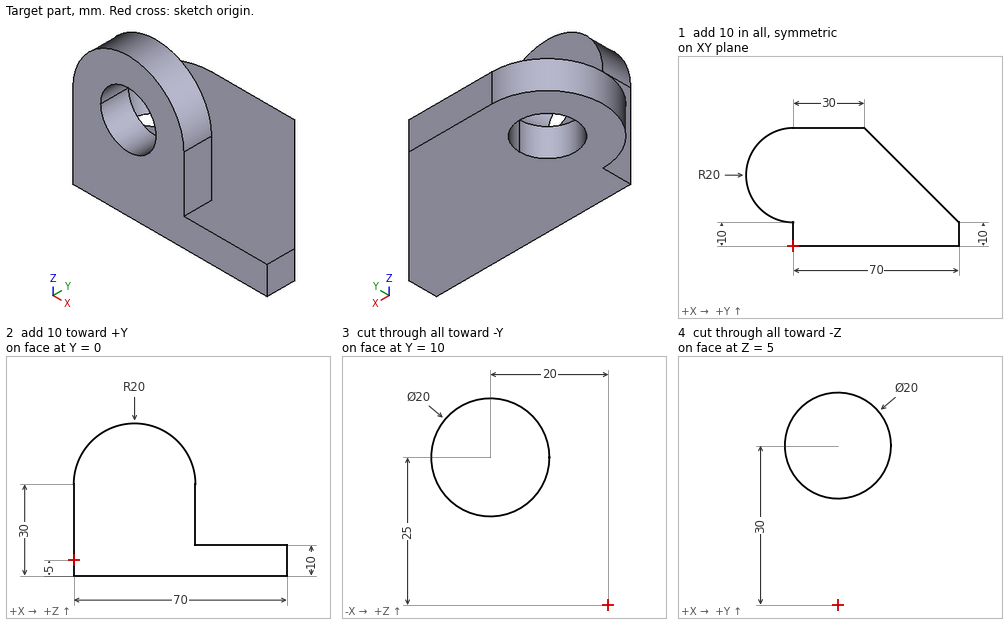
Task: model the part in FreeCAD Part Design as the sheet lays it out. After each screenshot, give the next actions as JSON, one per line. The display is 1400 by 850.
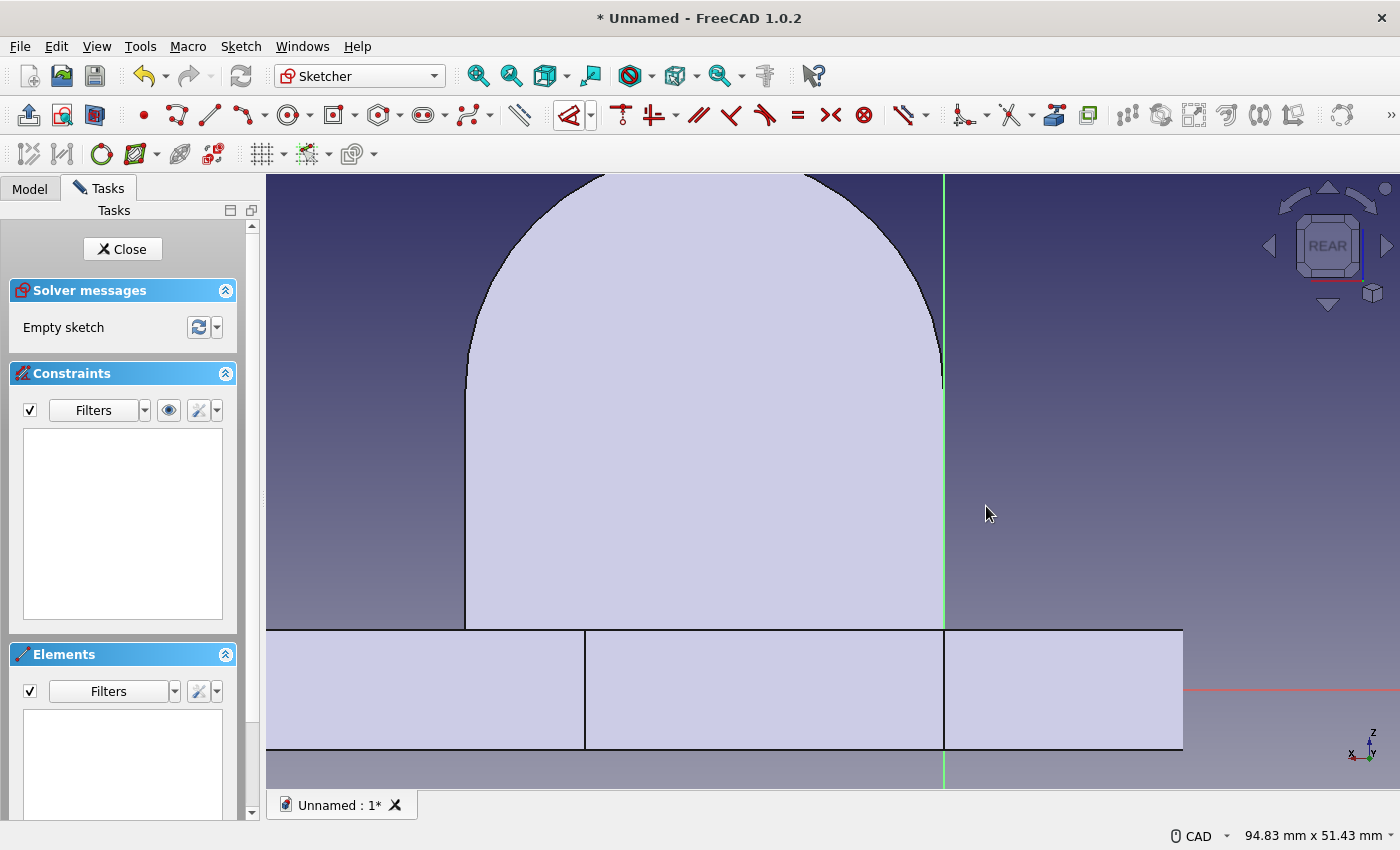
{"action": "left_click", "coordinate": [288, 116]}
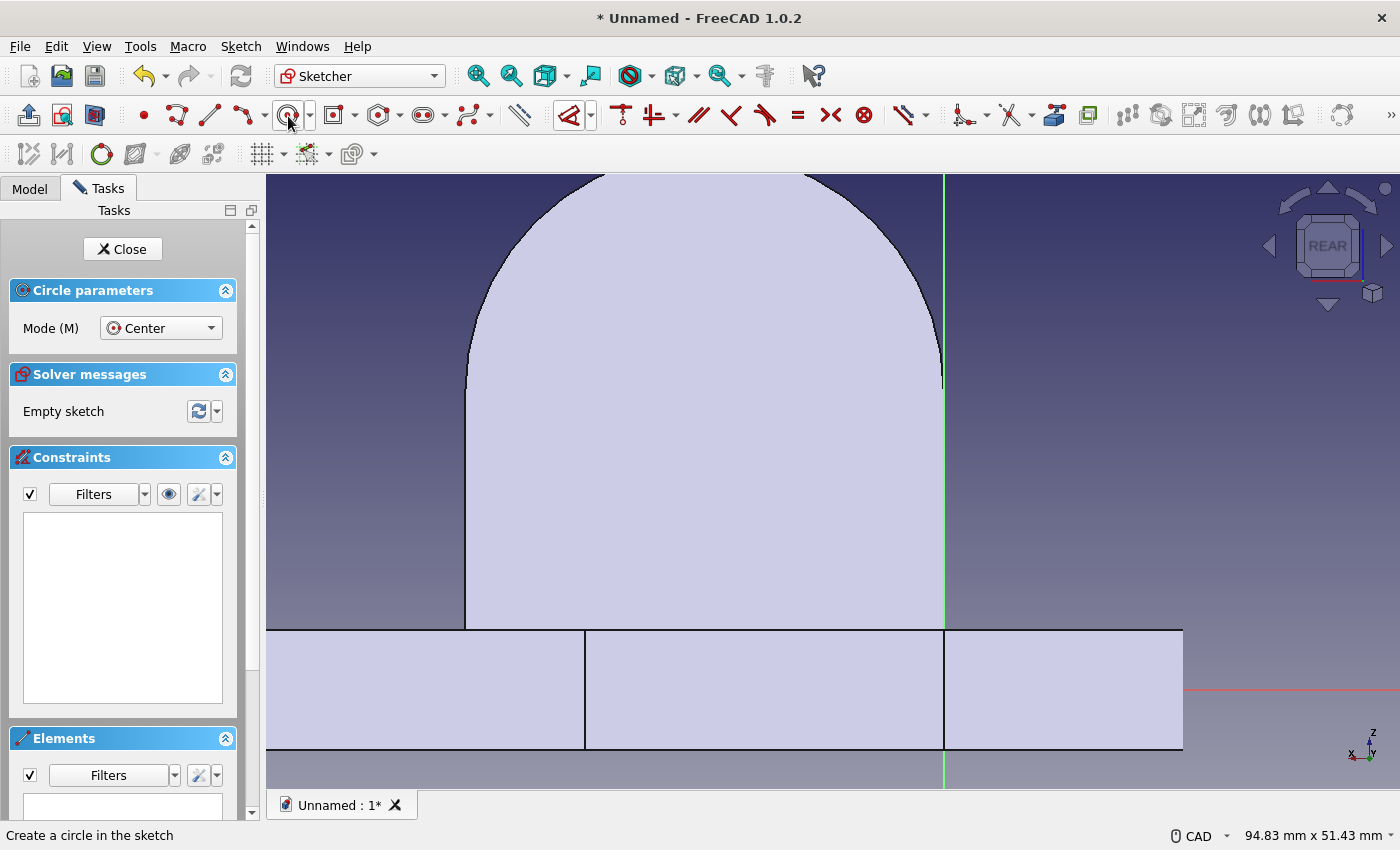
{"action": "left_click", "coordinate": [705, 391]}
{"action": "left_click", "coordinate": [789, 306]}
{"action": "key", "text": "Escape"}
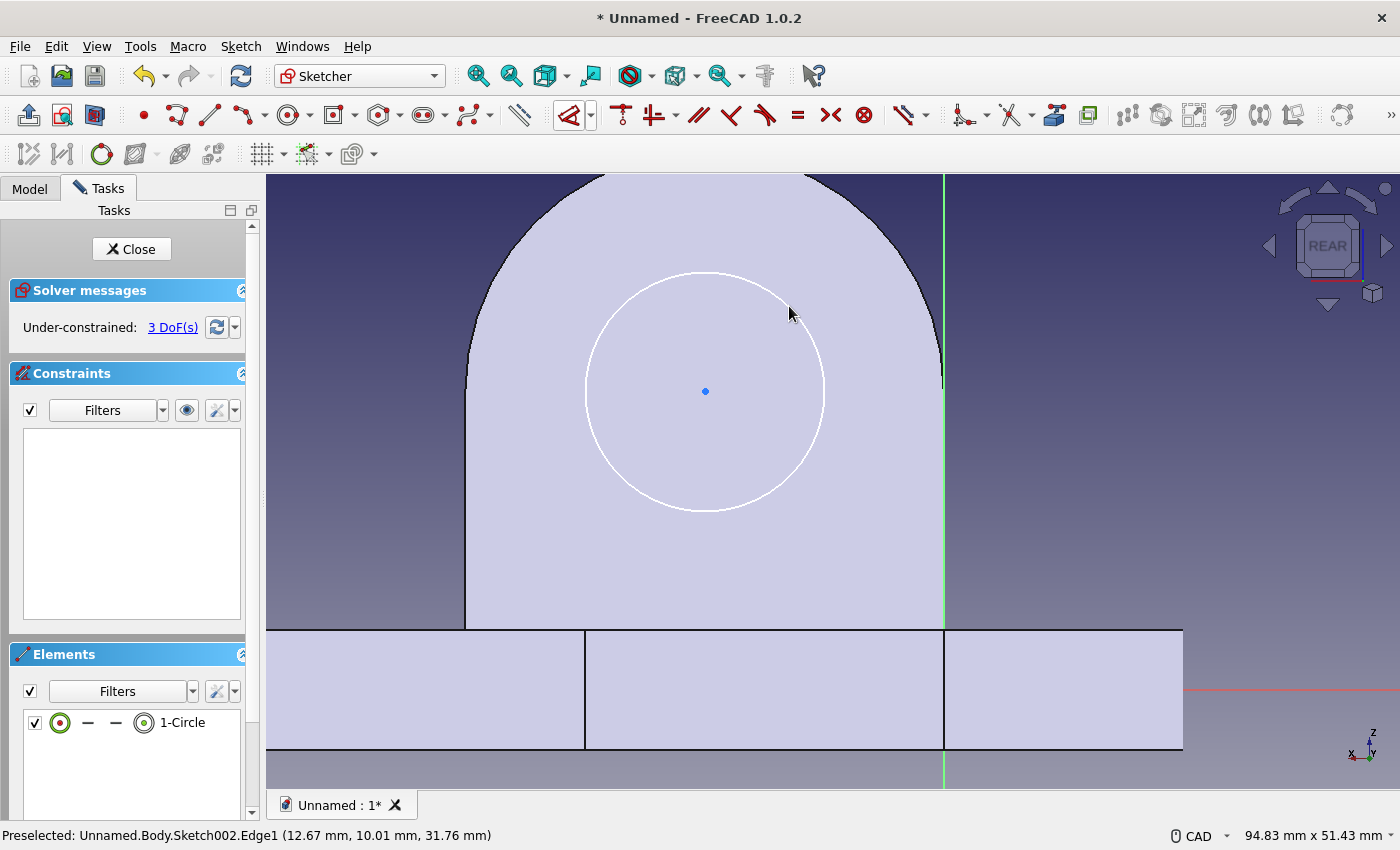
{"action": "left_click", "coordinate": [789, 307]}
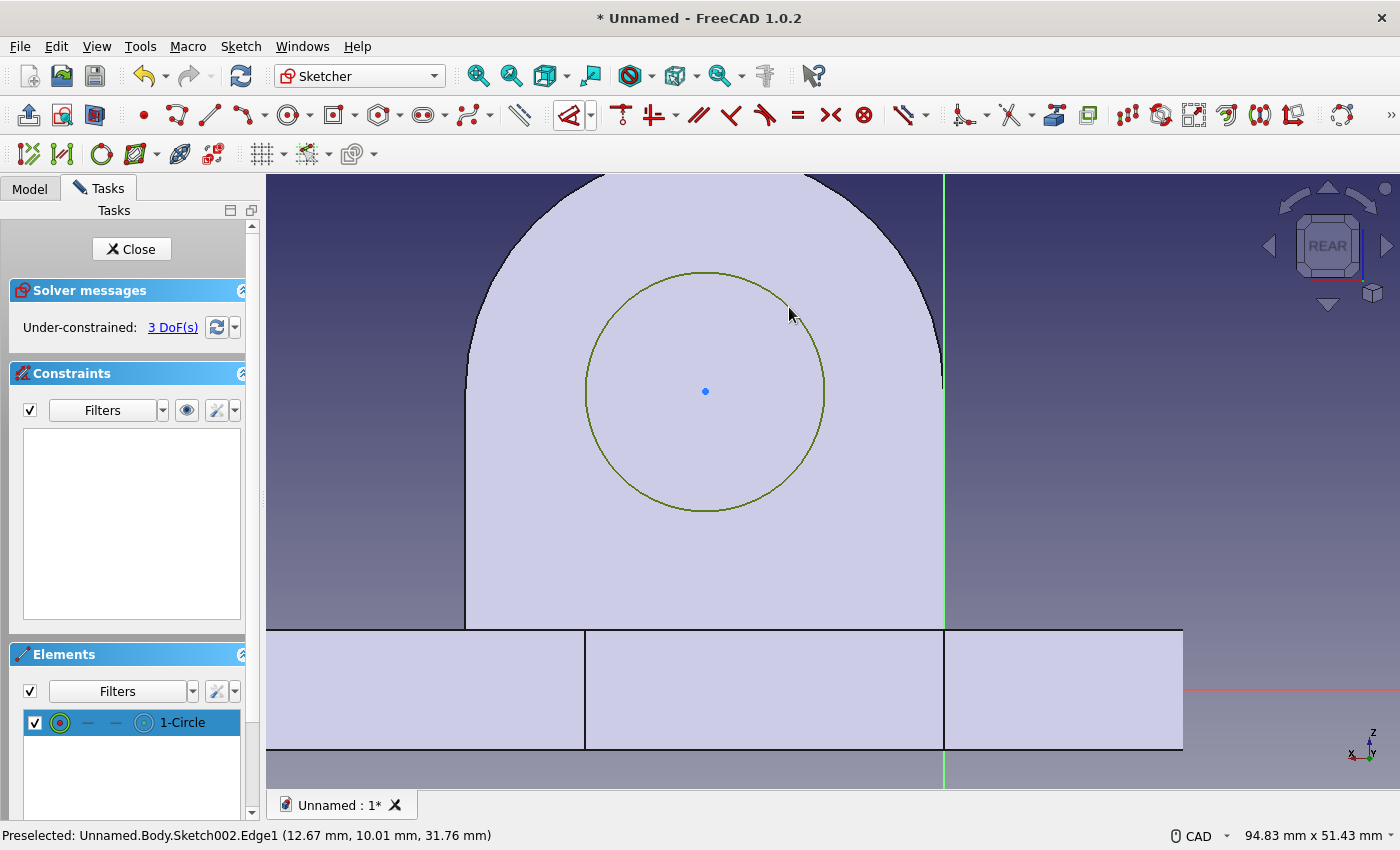
{"action": "left_click", "coordinate": [590, 116]}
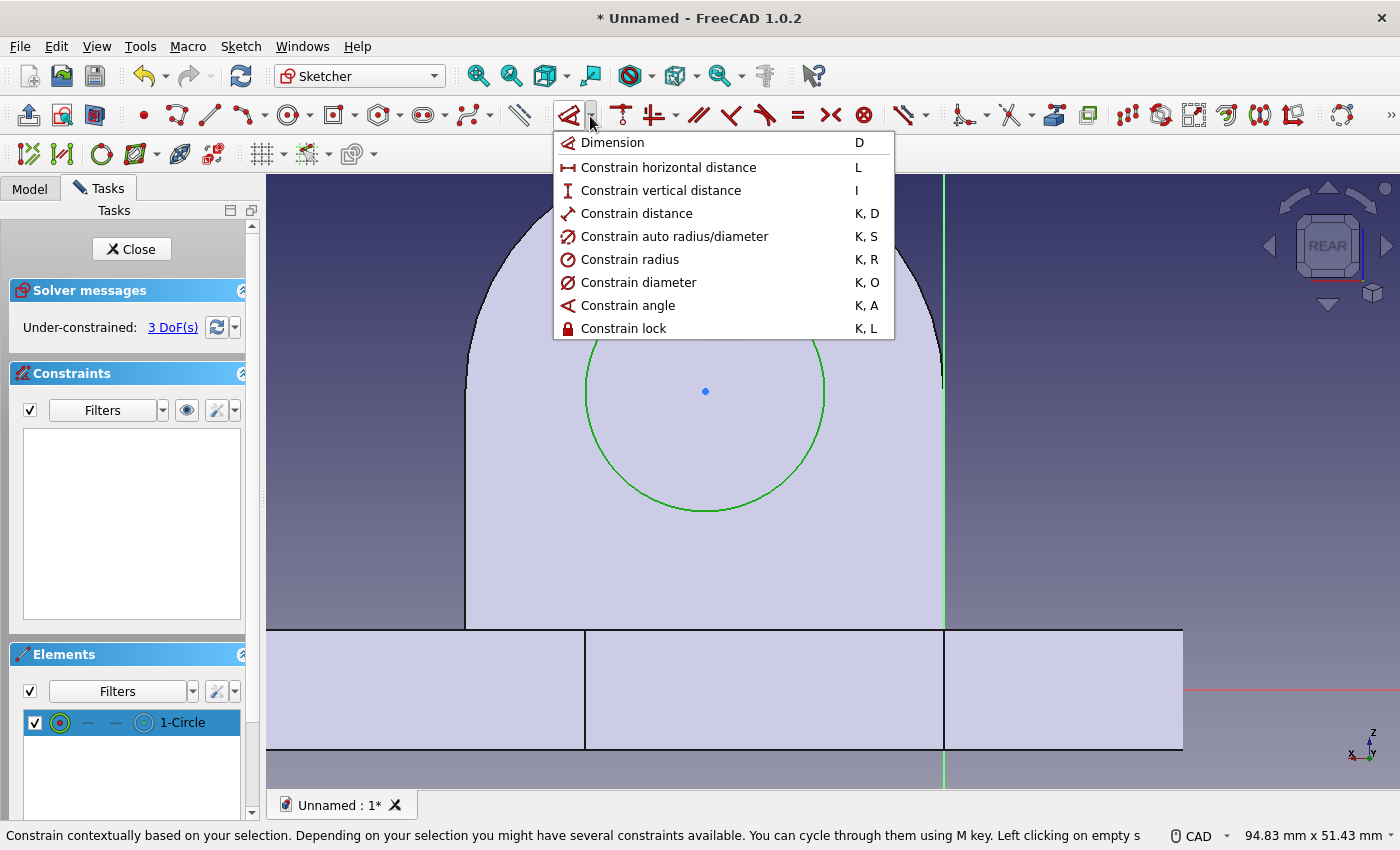
{"action": "left_click", "coordinate": [724, 282]}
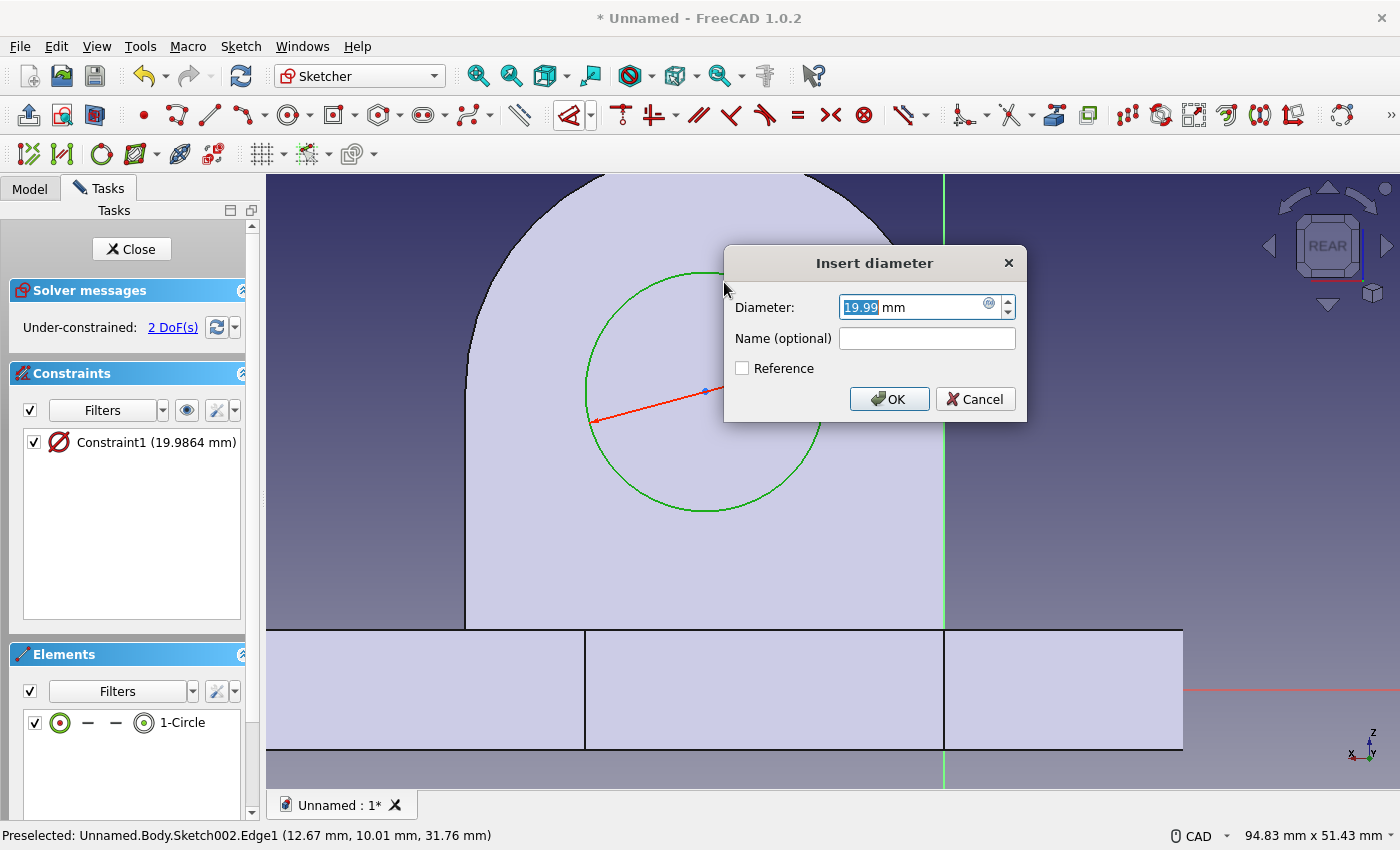
{"action": "type", "text": "20"}
{"action": "key", "text": "Return"}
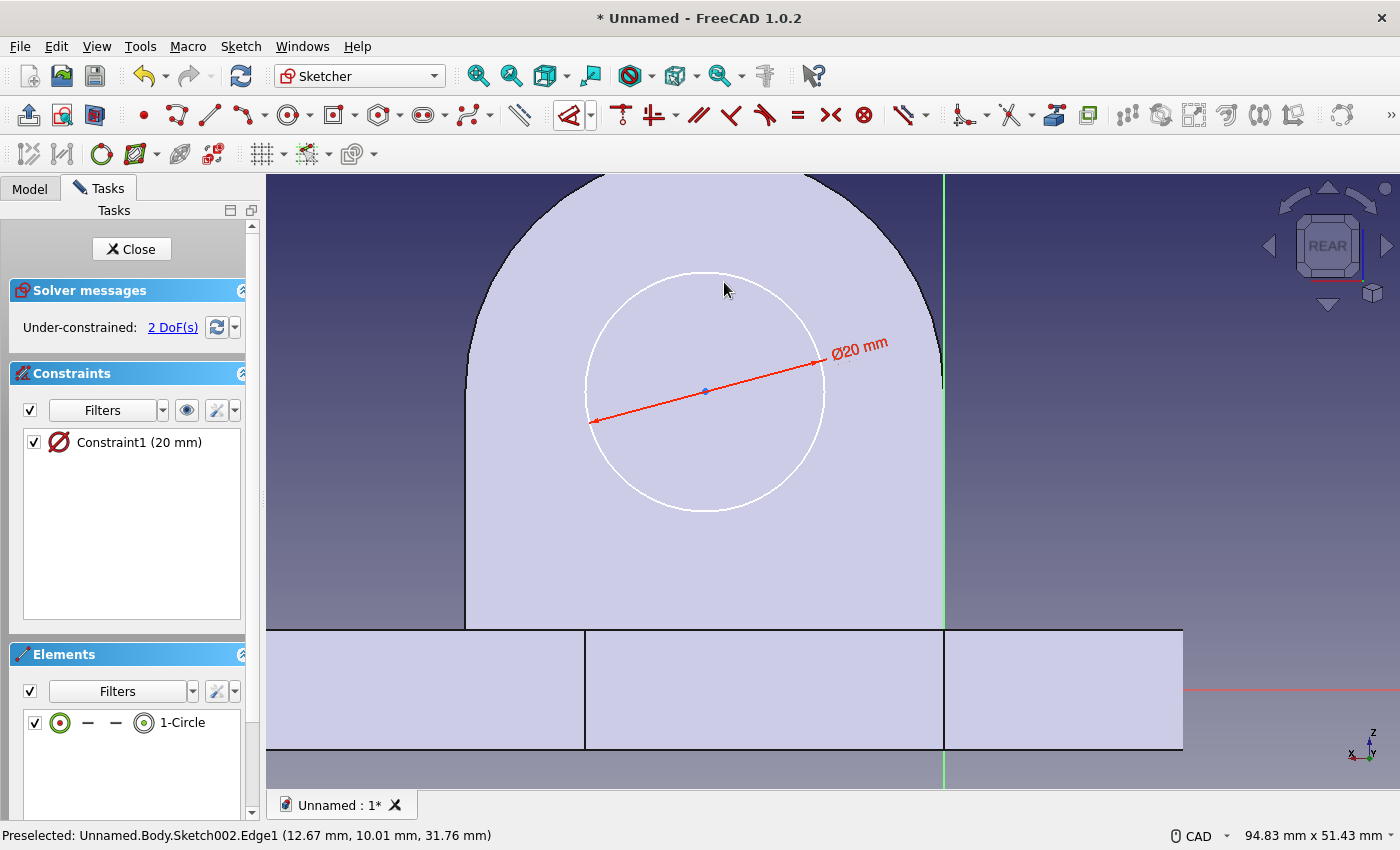
{"action": "left_click", "coordinate": [705, 392]}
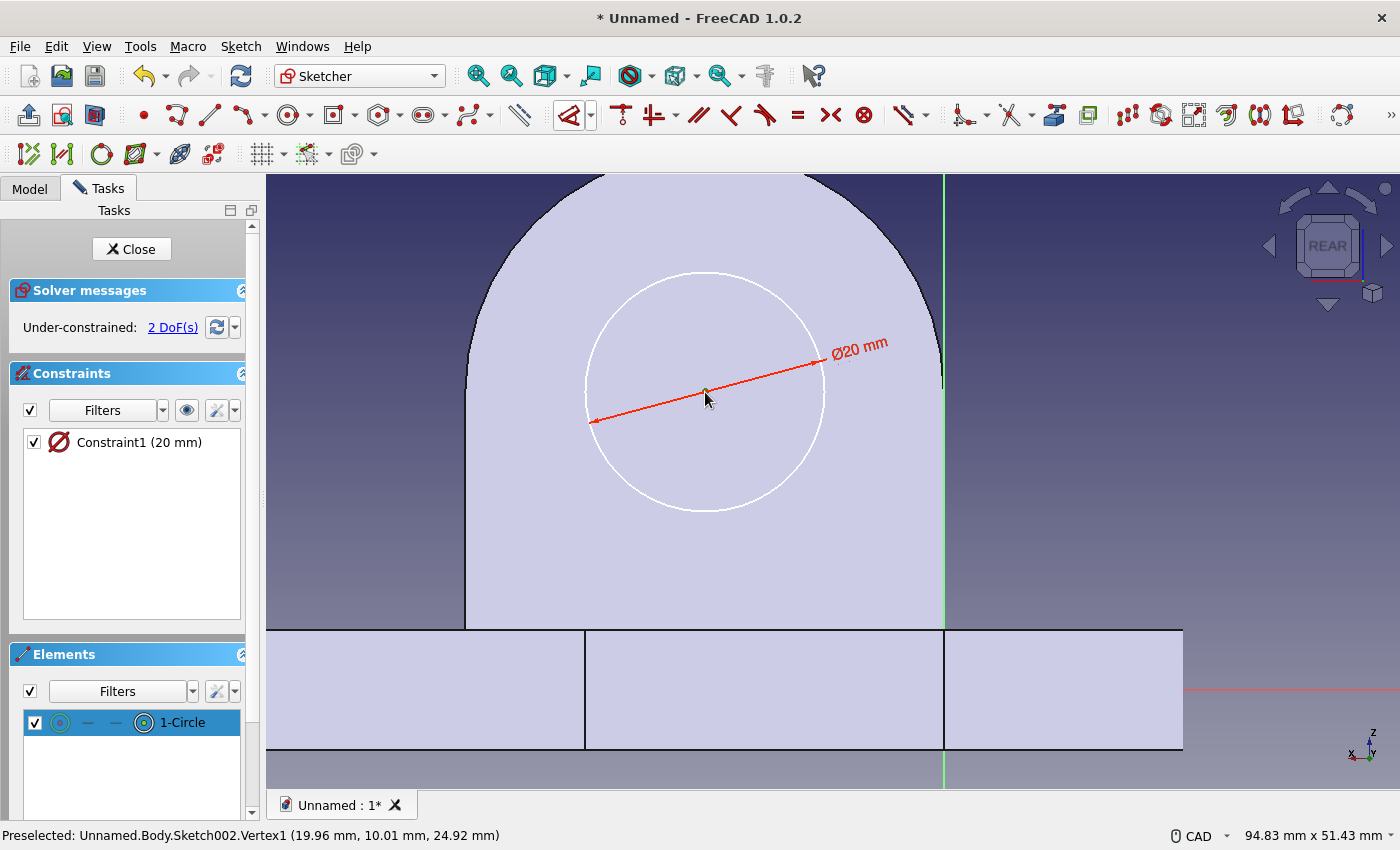
{"action": "key", "text": "l"}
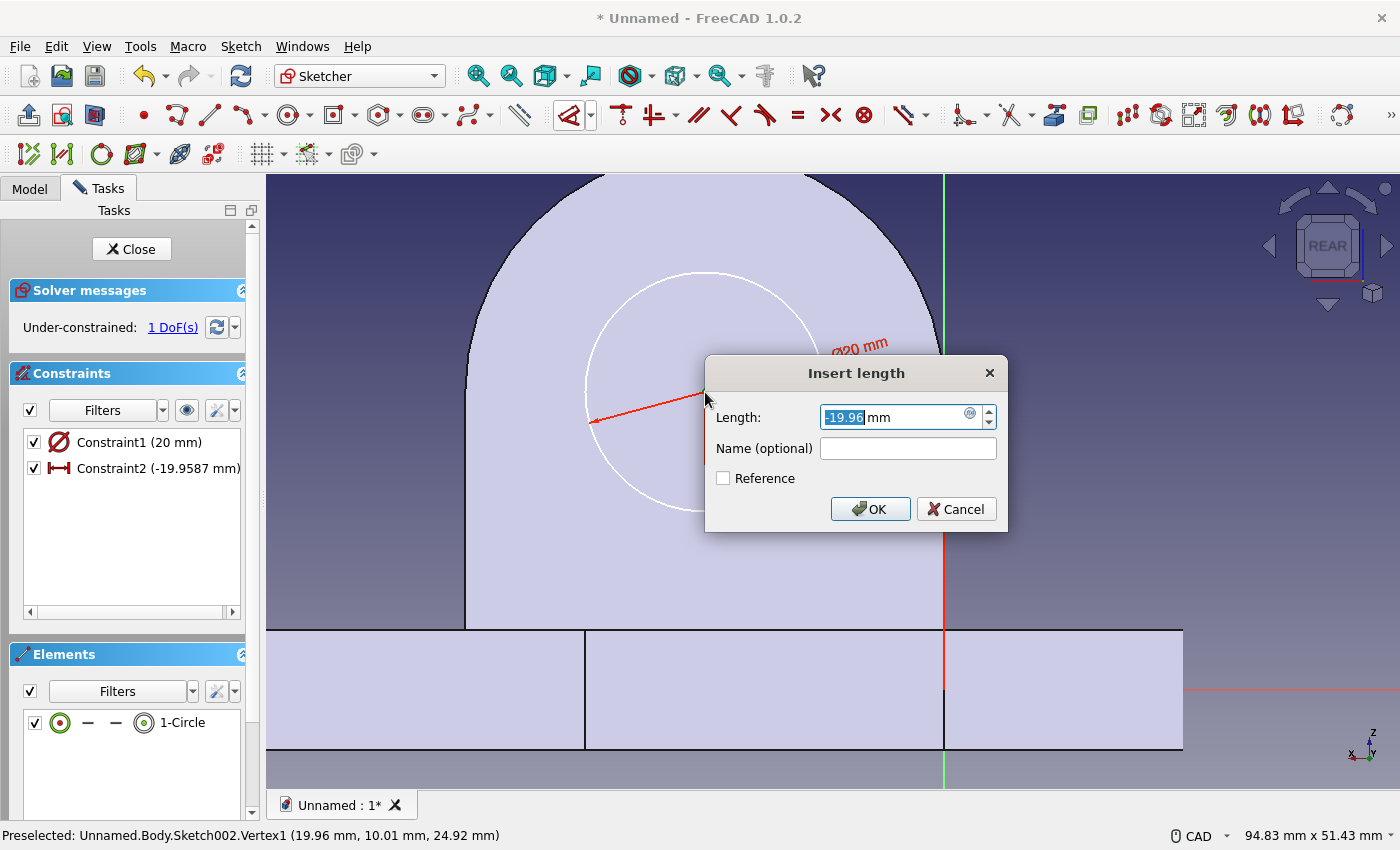
{"action": "type", "text": "-20"}
{"action": "key", "text": "Return"}